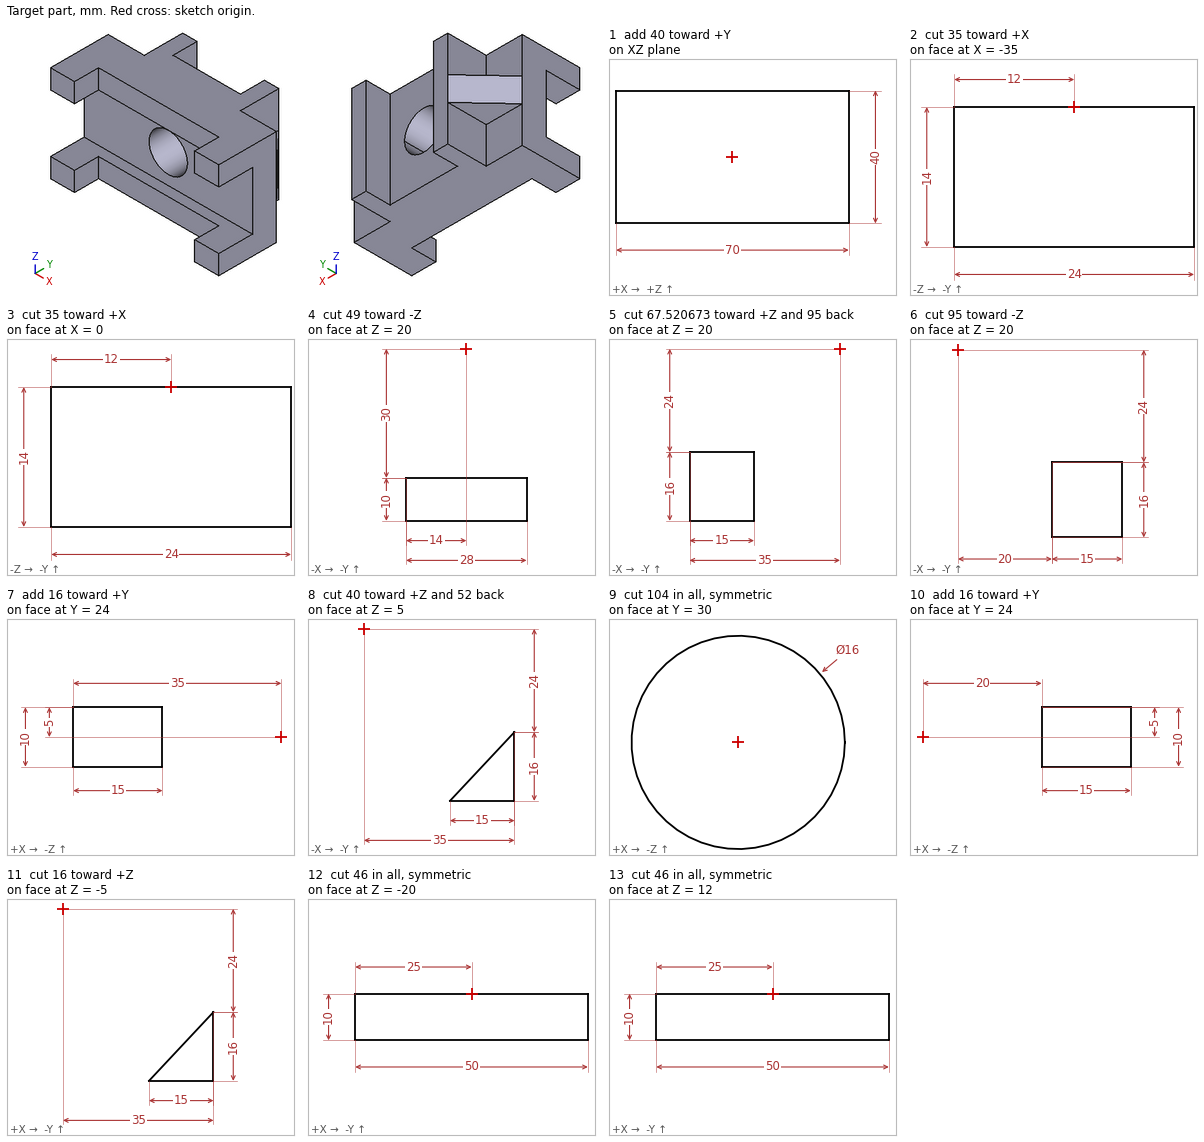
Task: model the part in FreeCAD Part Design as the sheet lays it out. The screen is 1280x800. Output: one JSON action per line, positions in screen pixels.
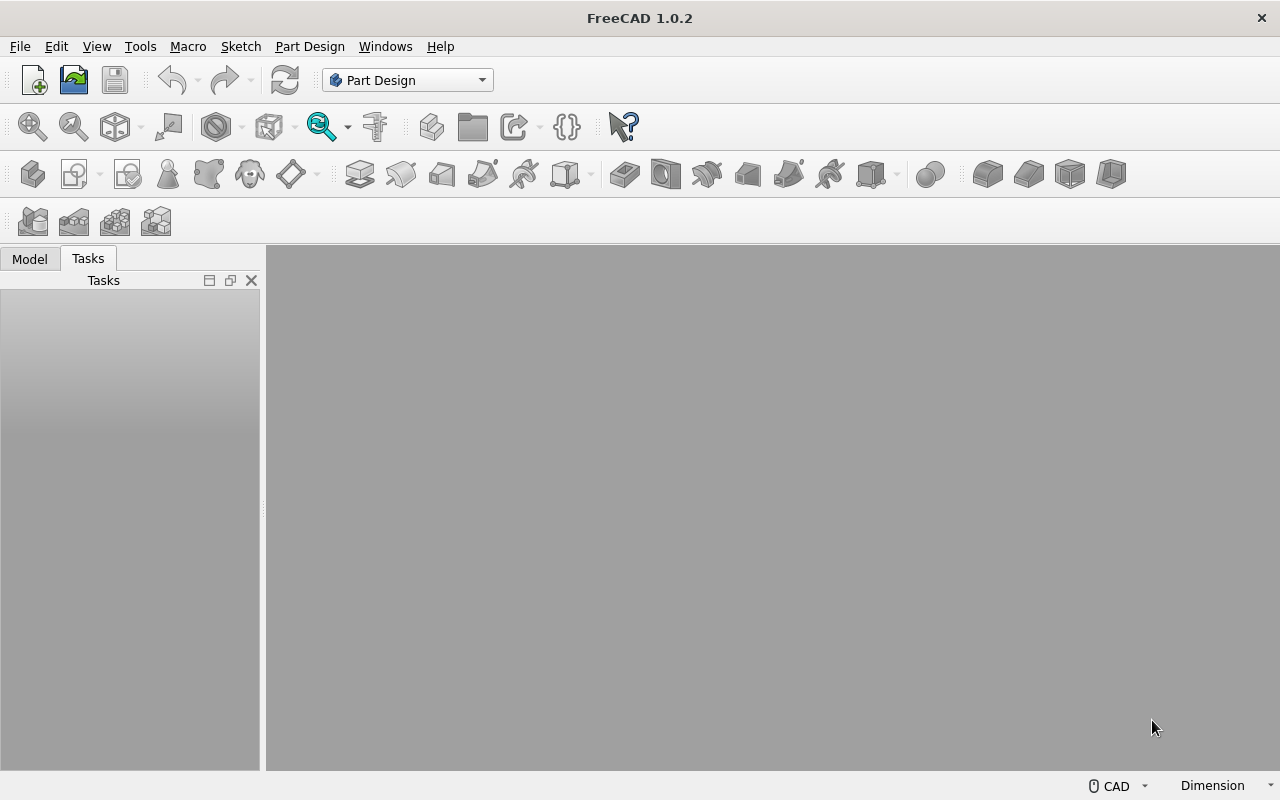
{"action": "key", "text": "ctrl+n"}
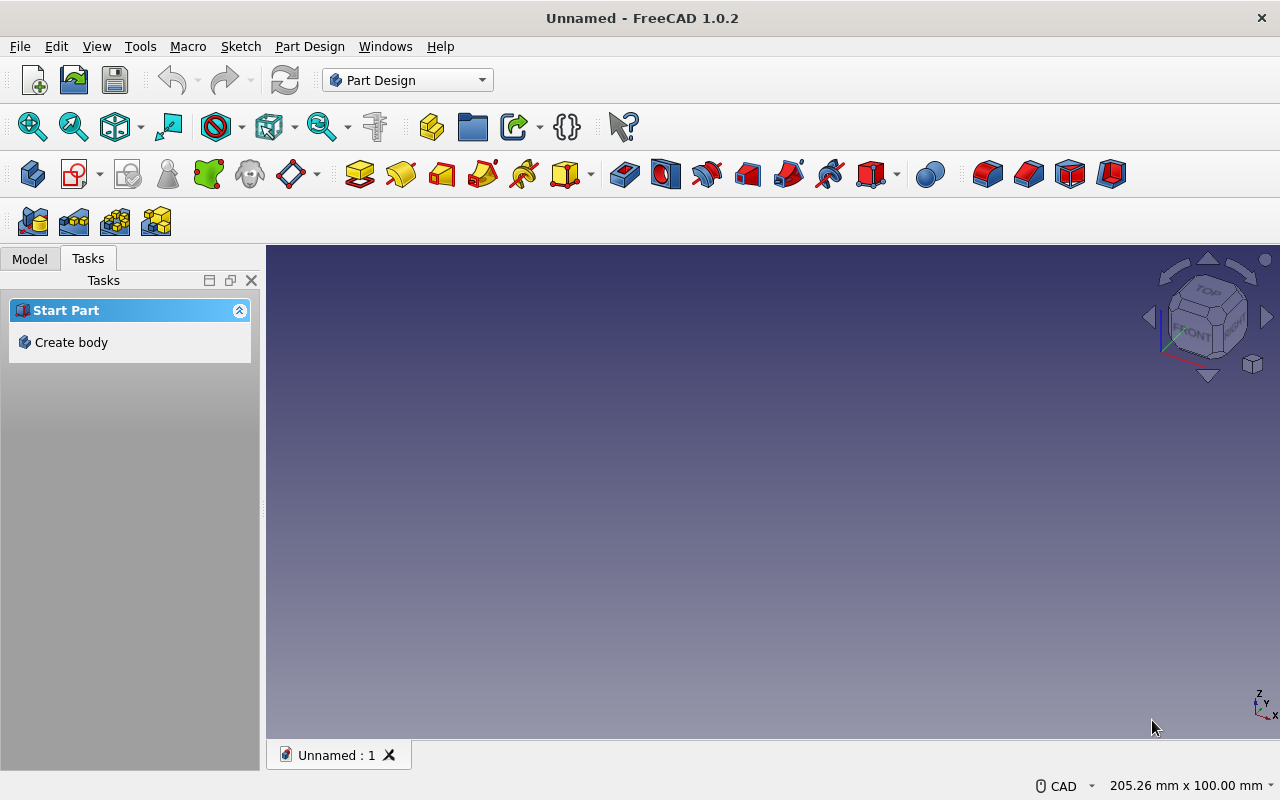
{"action": "left_click", "coordinate": [74, 174]}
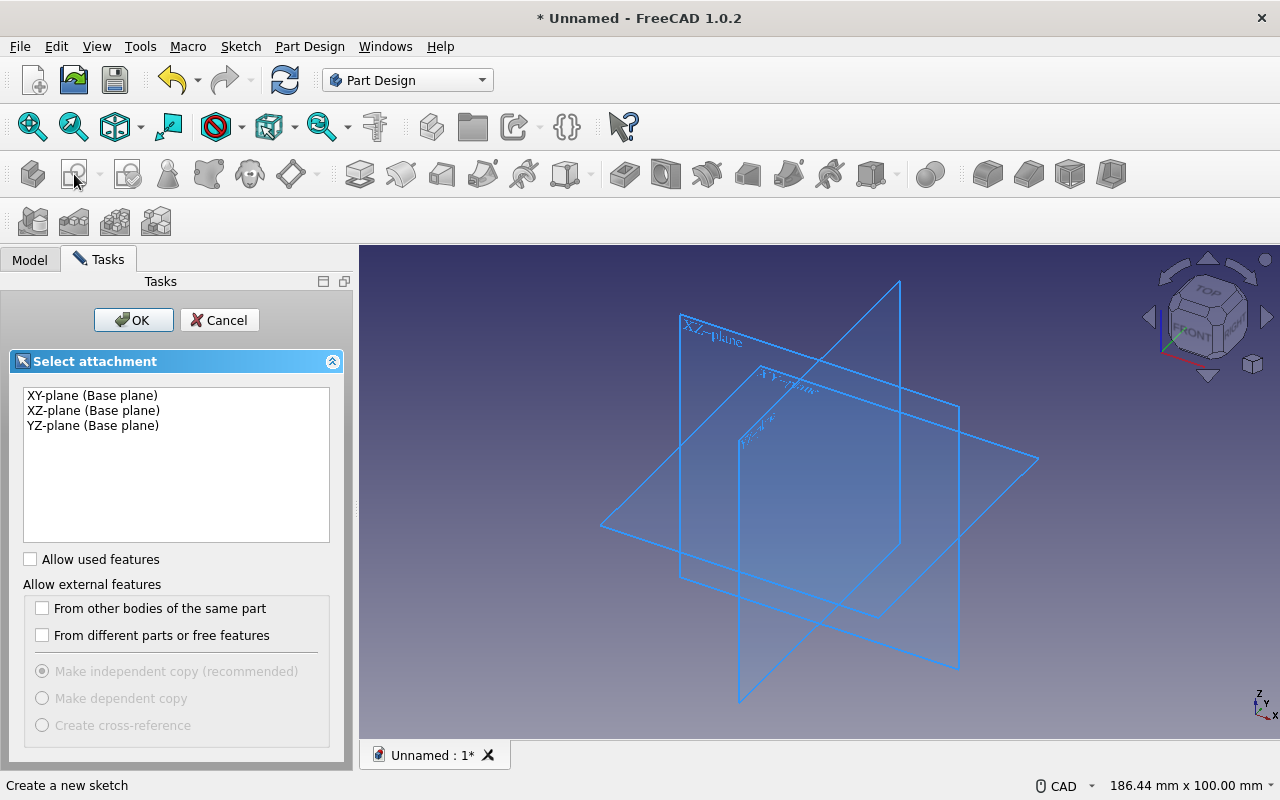
{"action": "left_click", "coordinate": [84, 410]}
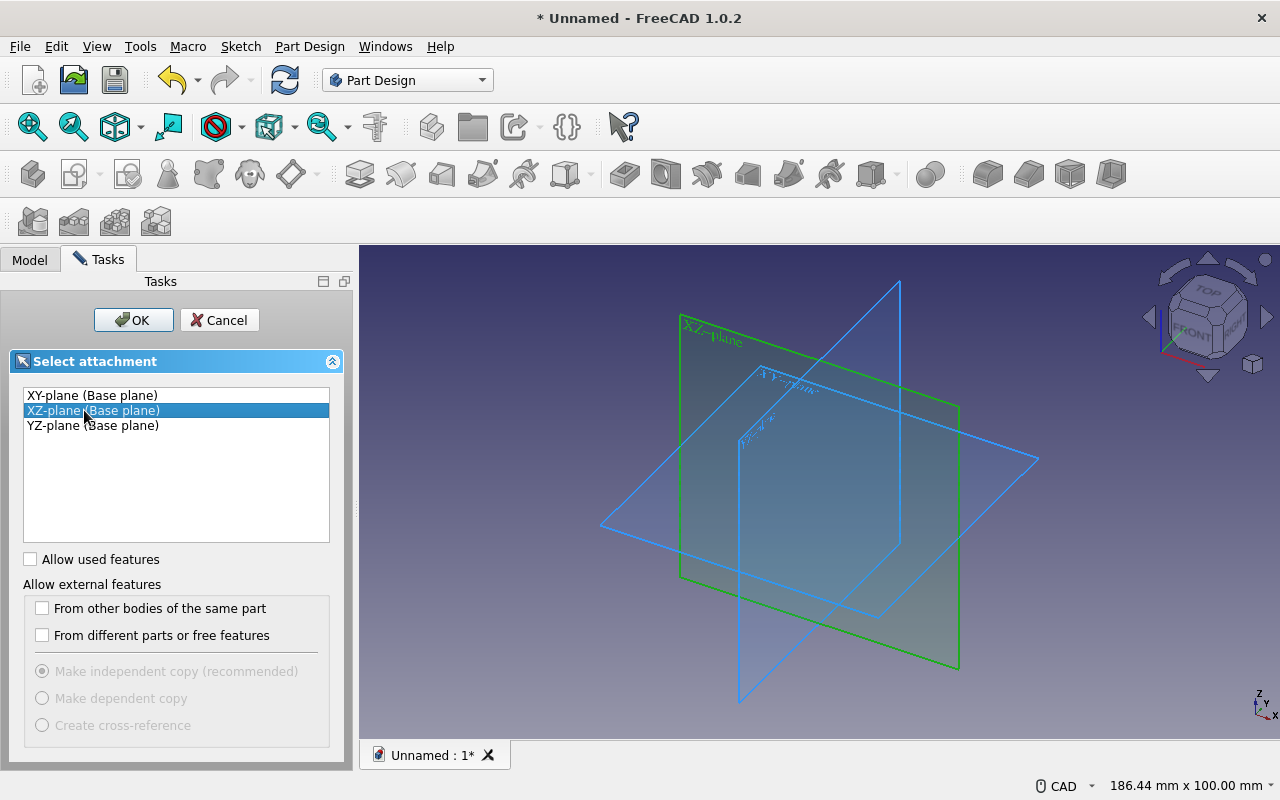
{"action": "left_click", "coordinate": [134, 320]}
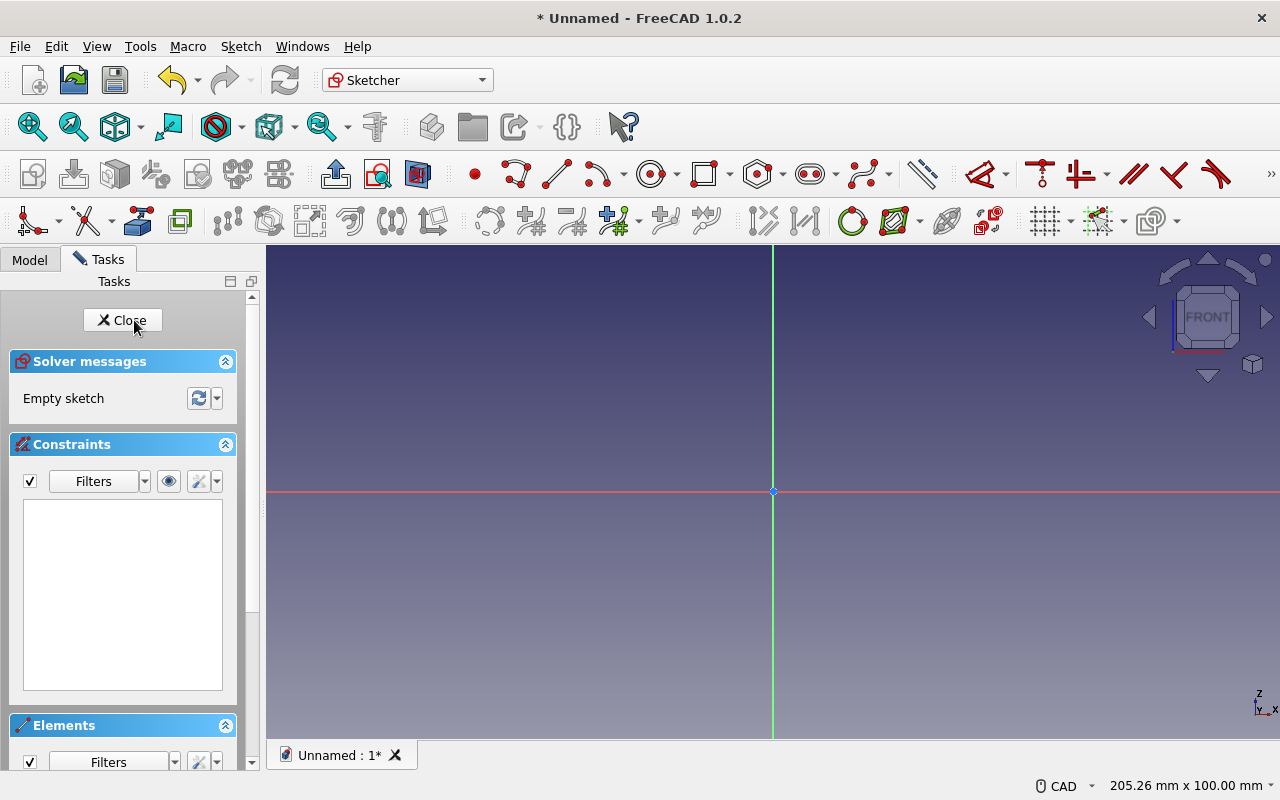
{"action": "scroll", "coordinate": [912, 492], "scroll_direction": "up", "scroll_amount": 2}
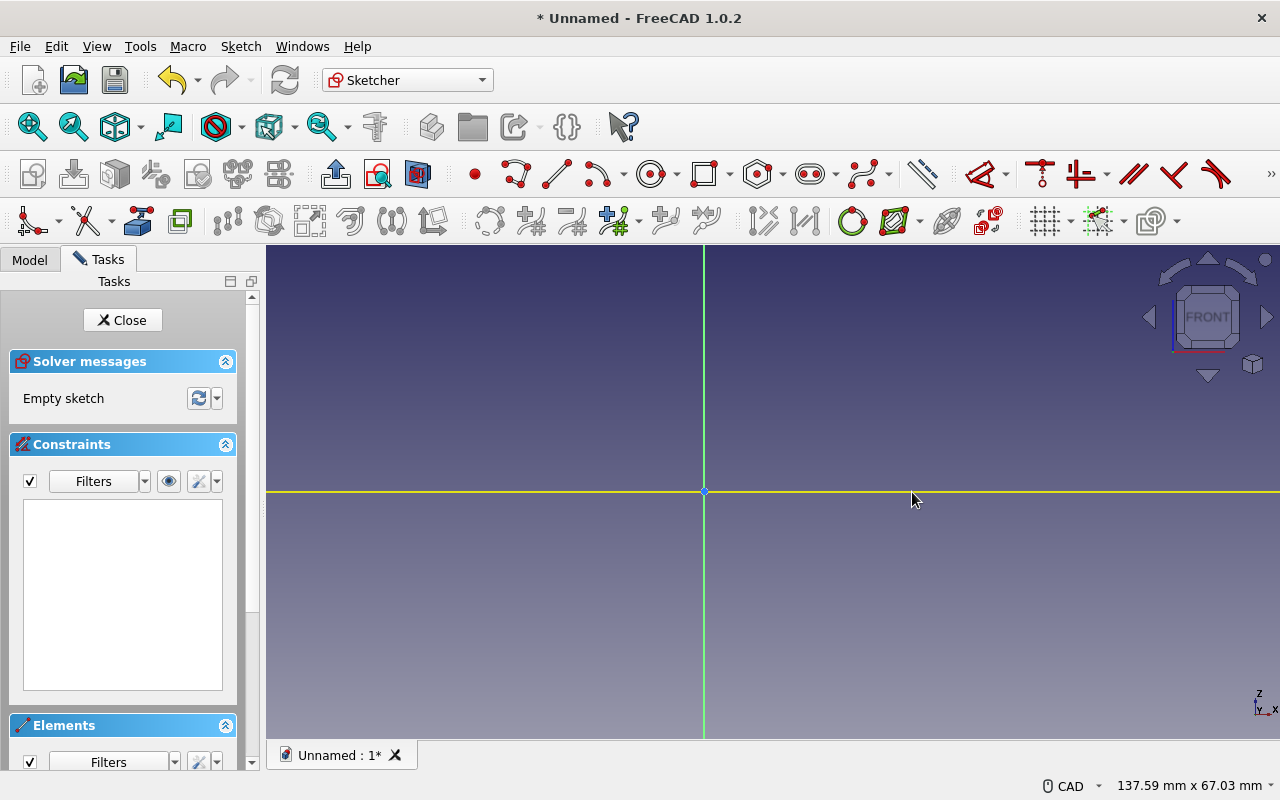
{"action": "left_click", "coordinate": [730, 174]}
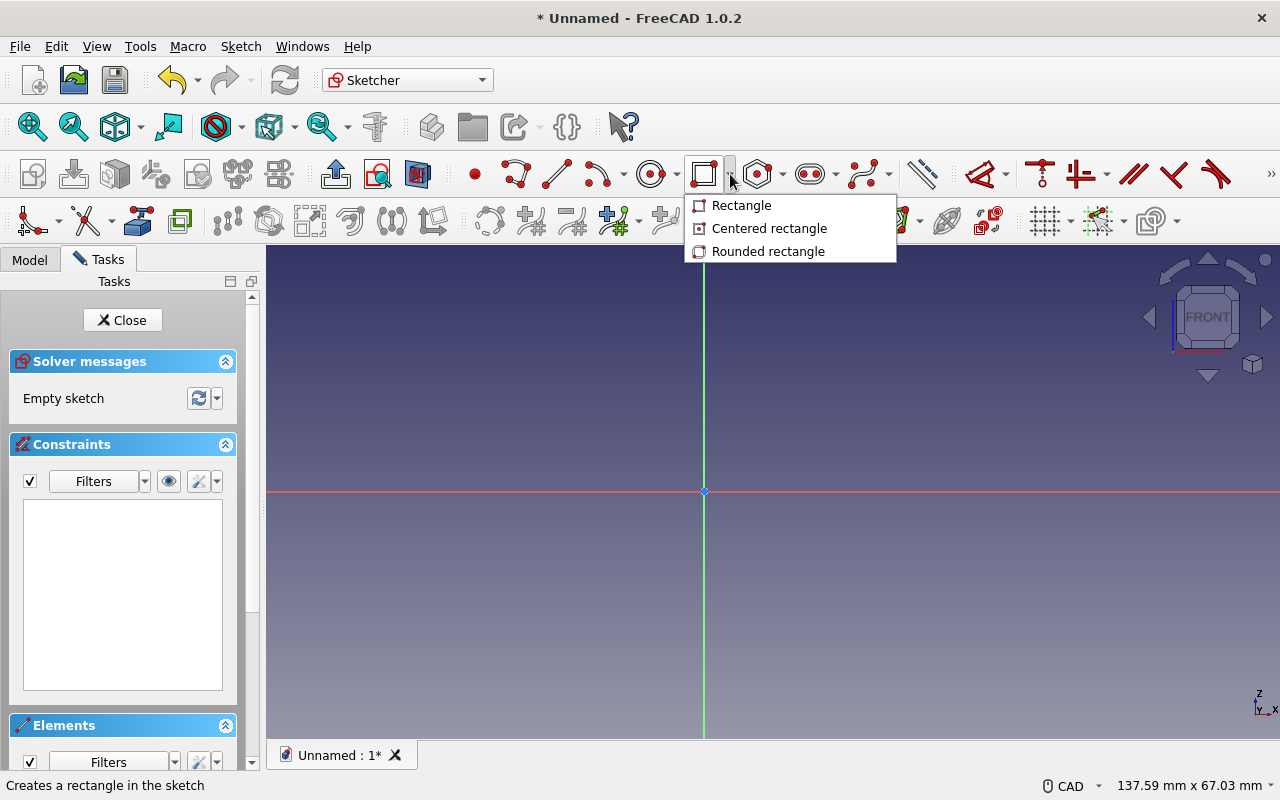
{"action": "left_click", "coordinate": [790, 228]}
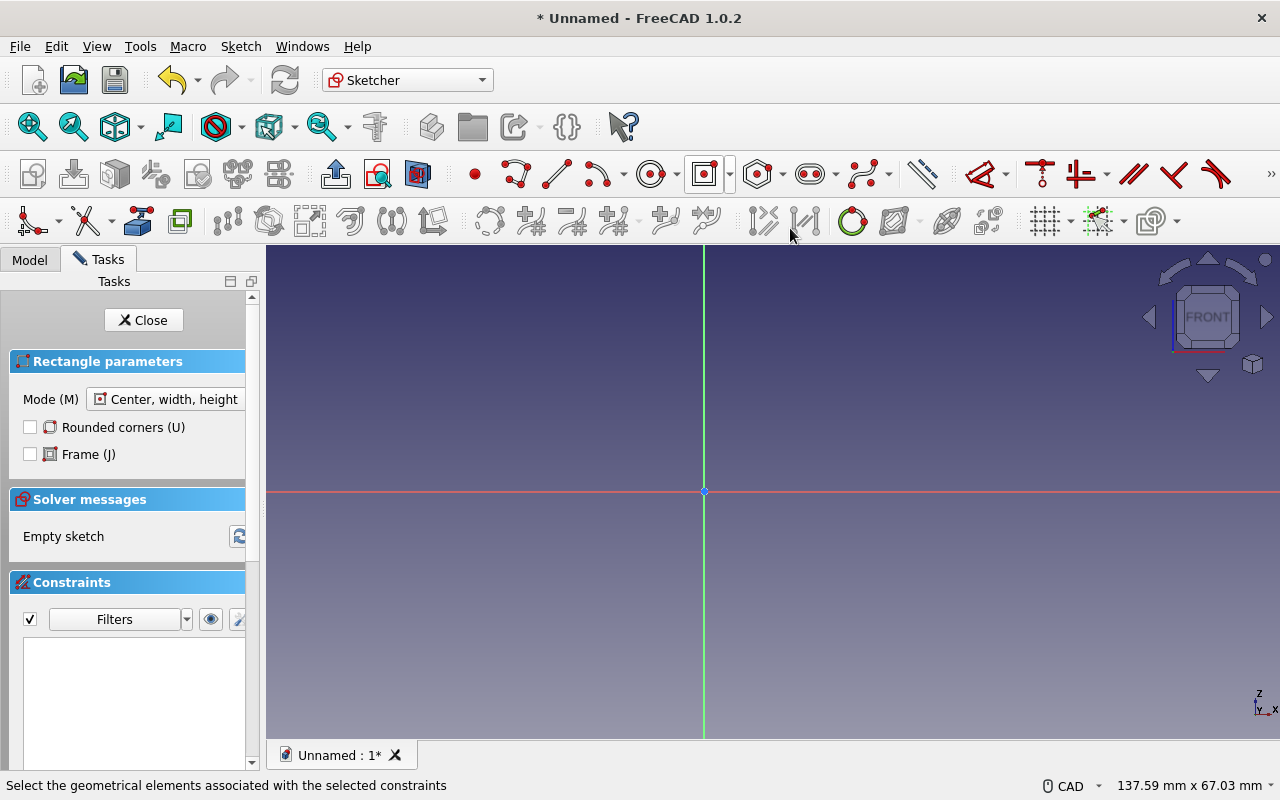
{"action": "left_click", "coordinate": [704, 492]}
{"action": "left_click", "coordinate": [962, 344]}
{"action": "key", "text": "Escape"}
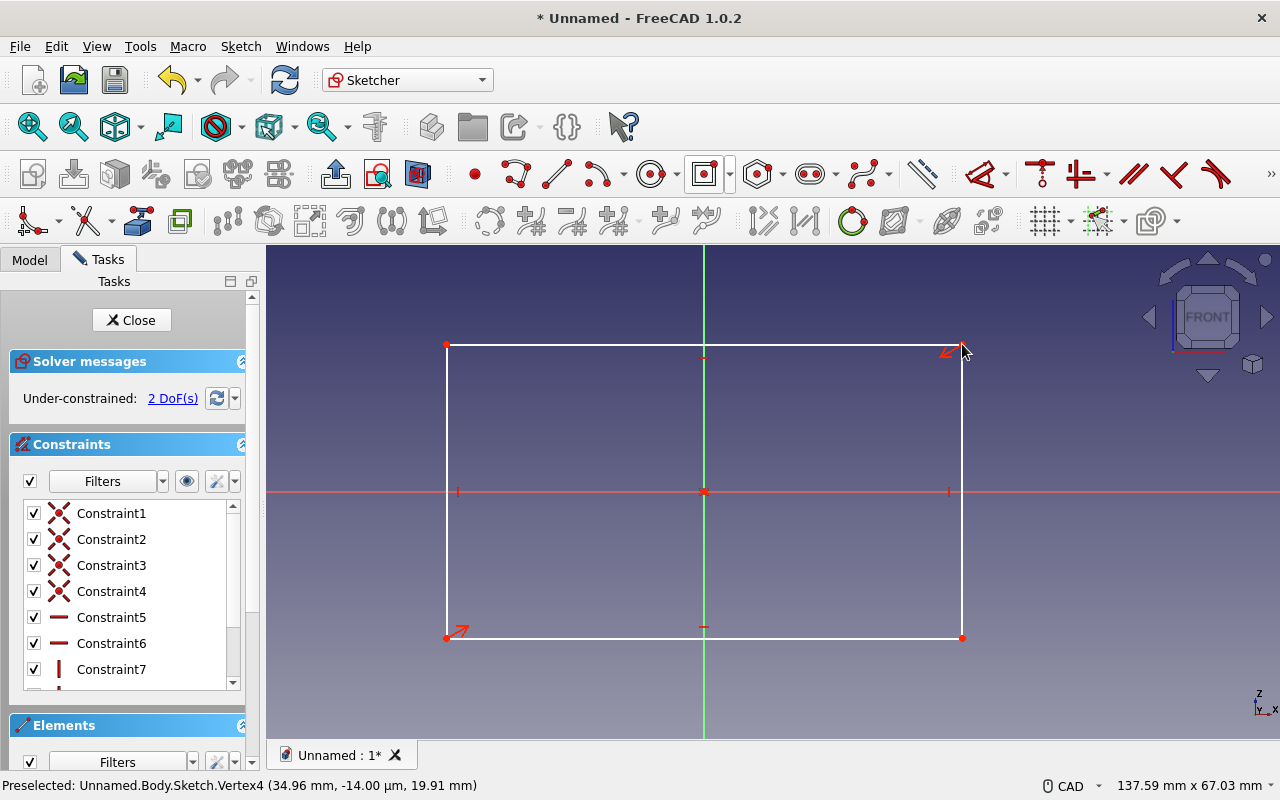
{"action": "left_click", "coordinate": [601, 639]}